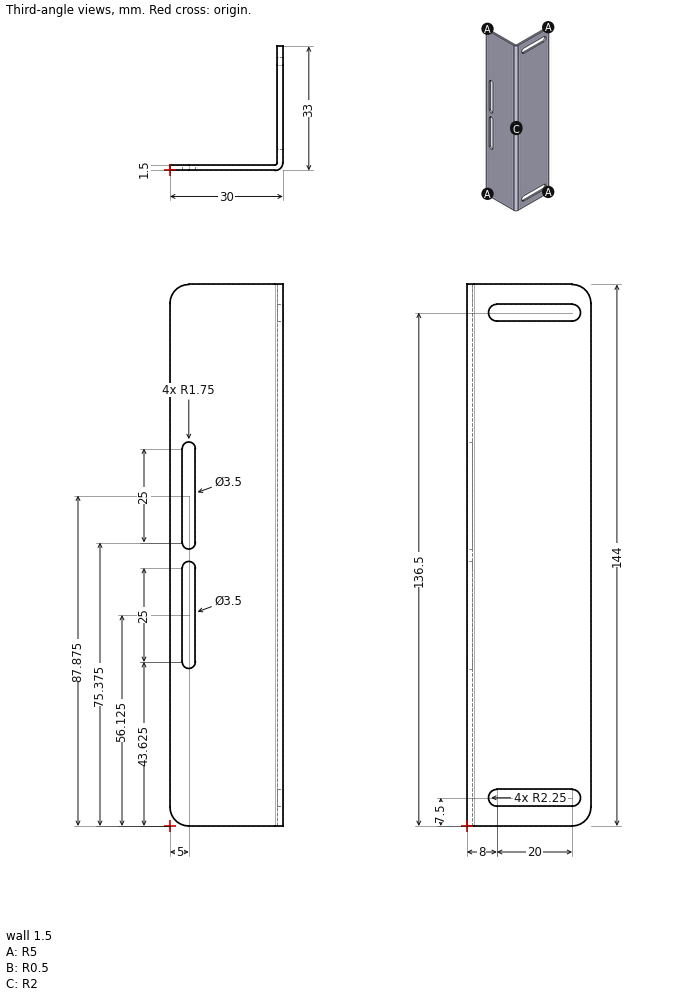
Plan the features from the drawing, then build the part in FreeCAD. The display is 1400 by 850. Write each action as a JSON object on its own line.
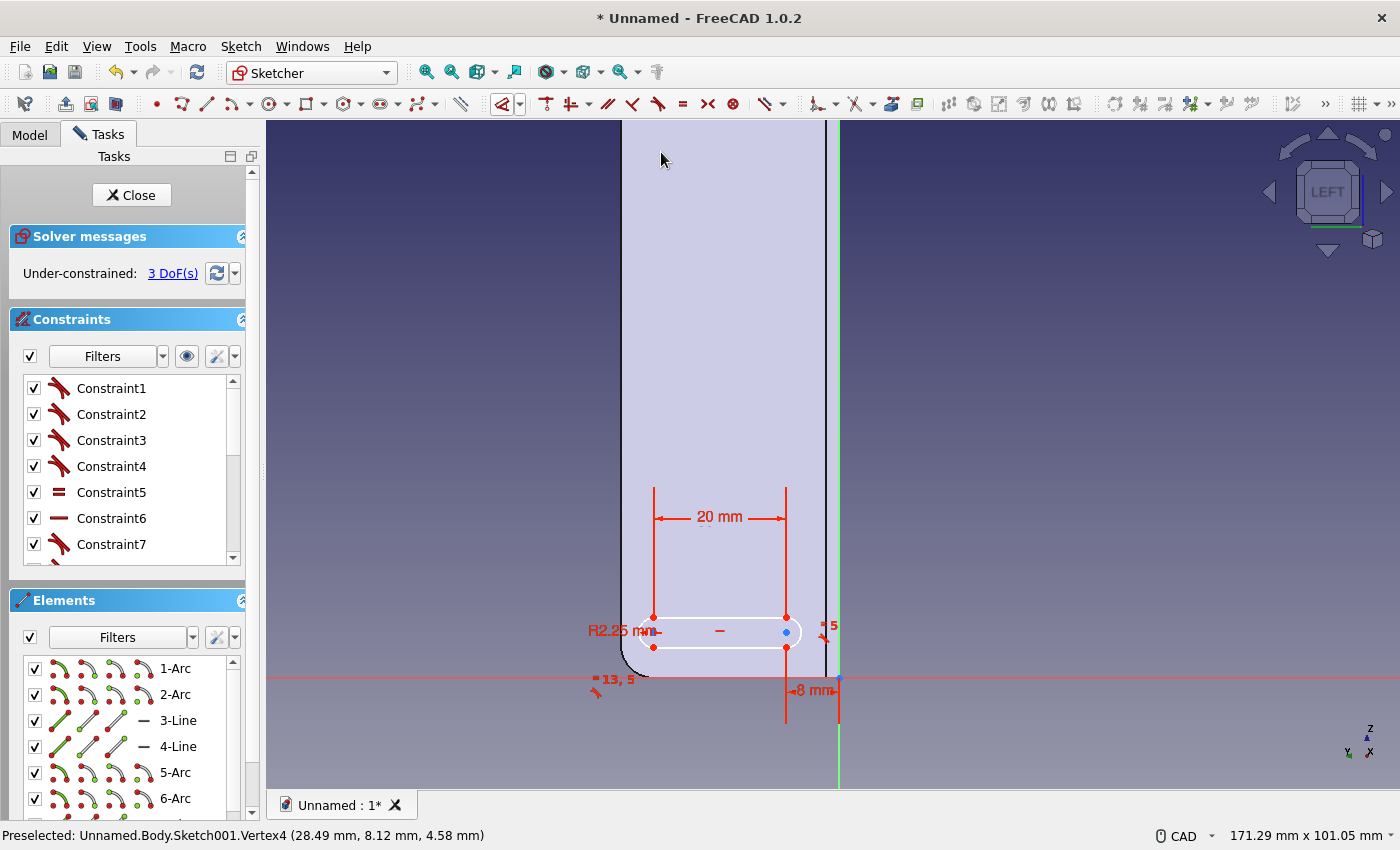
{"action": "scroll", "coordinate": [785, 647], "scroll_direction": "down", "scroll_amount": 4}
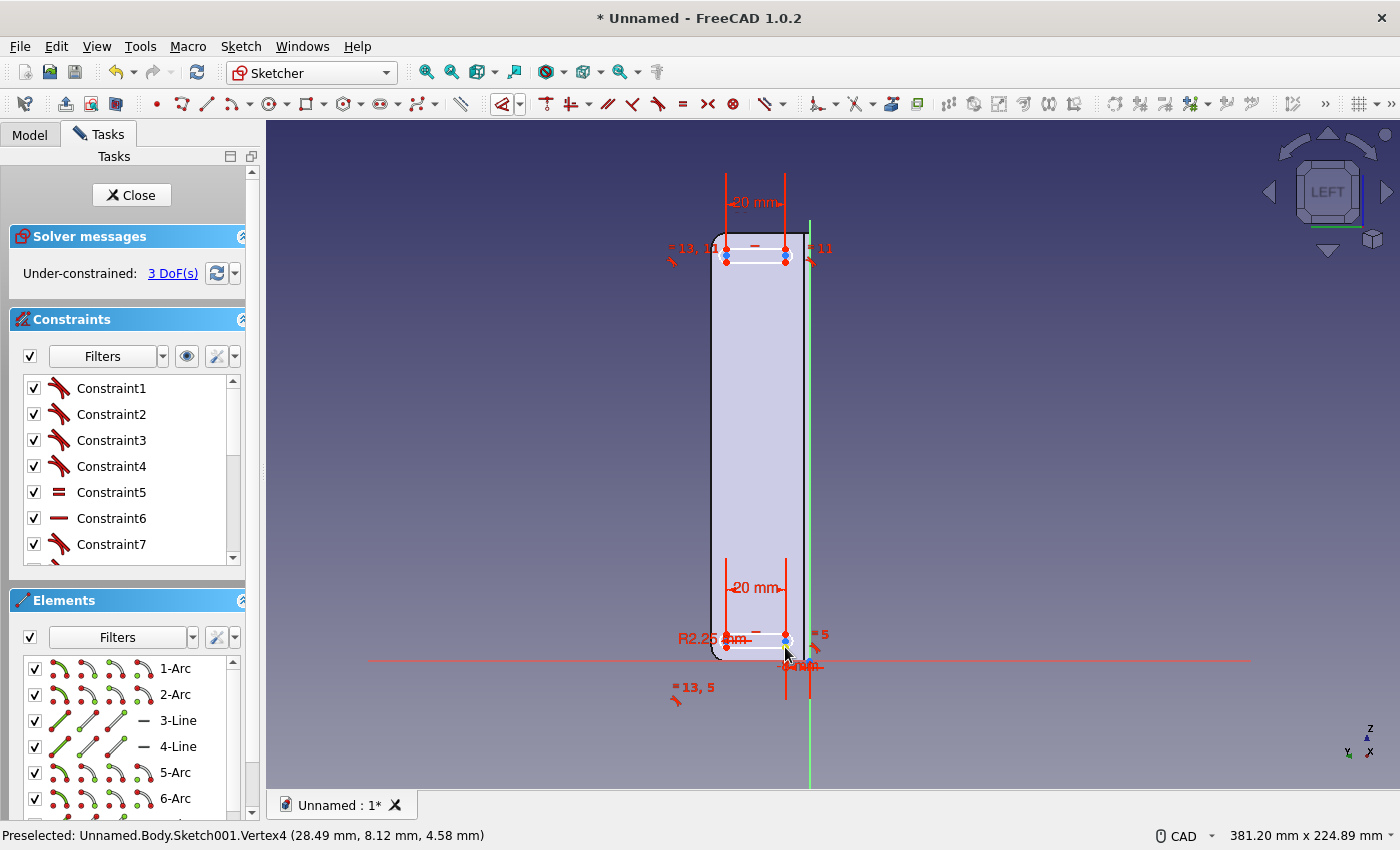
{"action": "scroll", "coordinate": [785, 263], "scroll_direction": "up", "scroll_amount": 4}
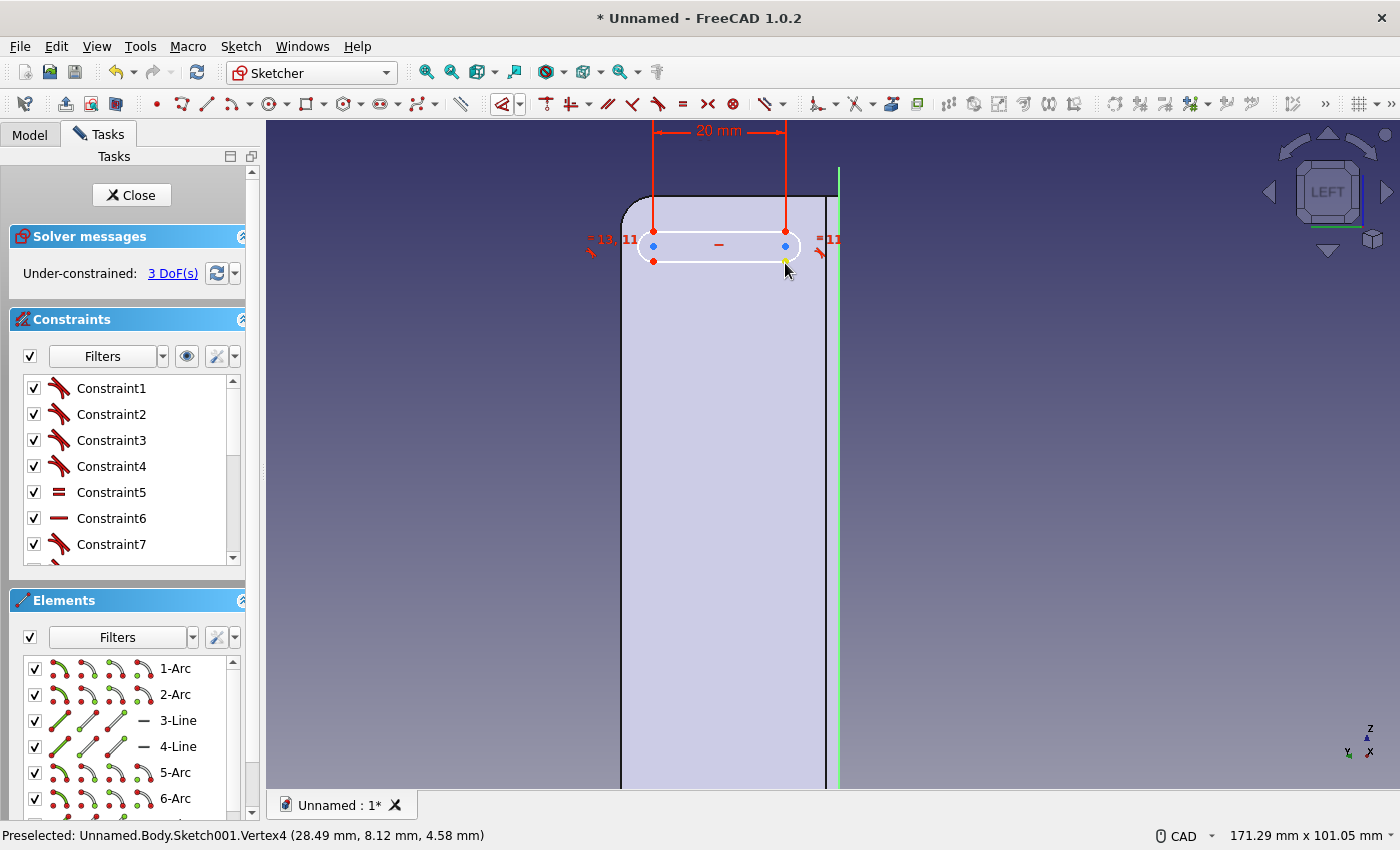
{"action": "left_click", "coordinate": [786, 262]}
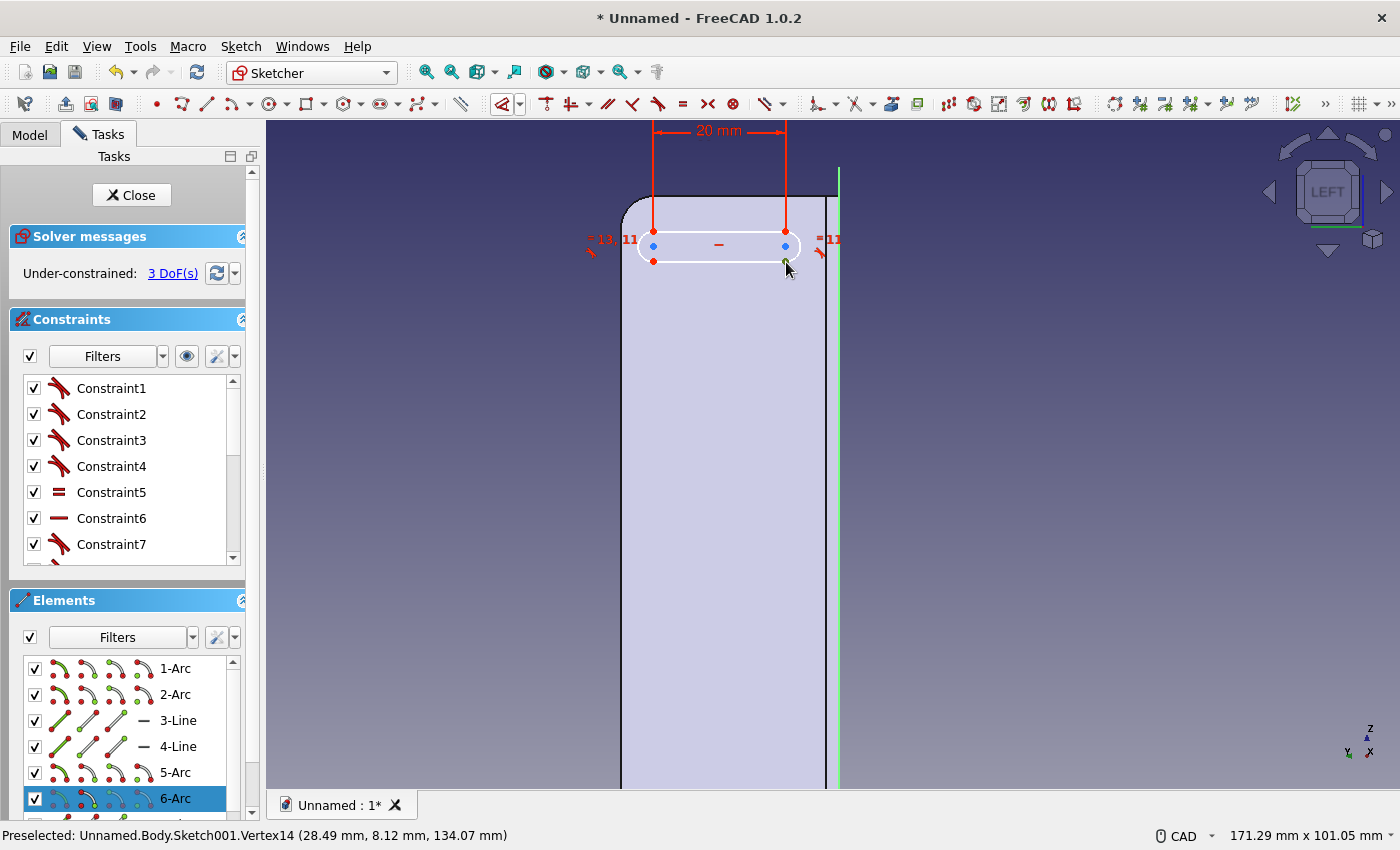
{"action": "key", "text": "l"}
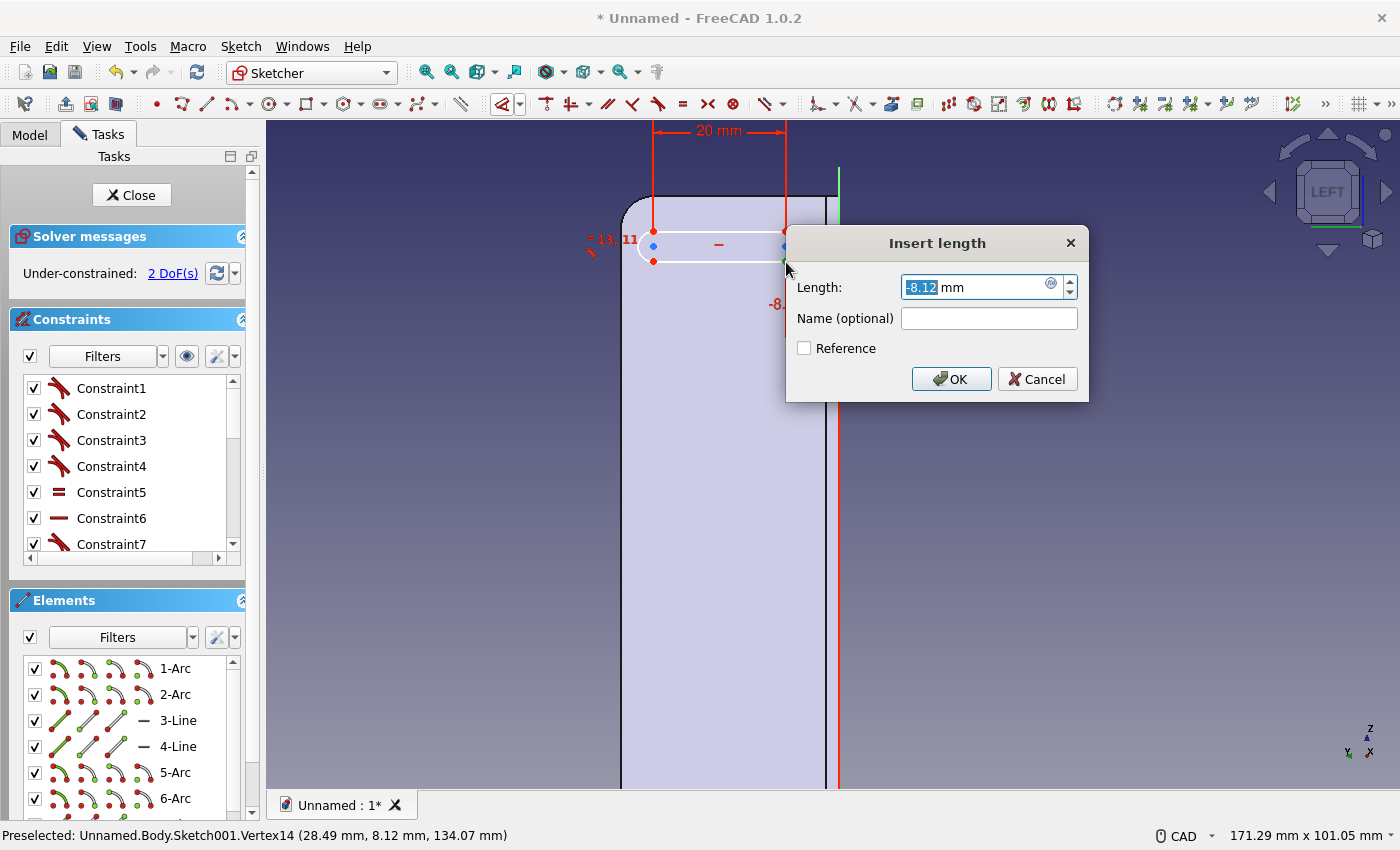
{"action": "type", "text": "-8"}
{"action": "key", "text": "Return"}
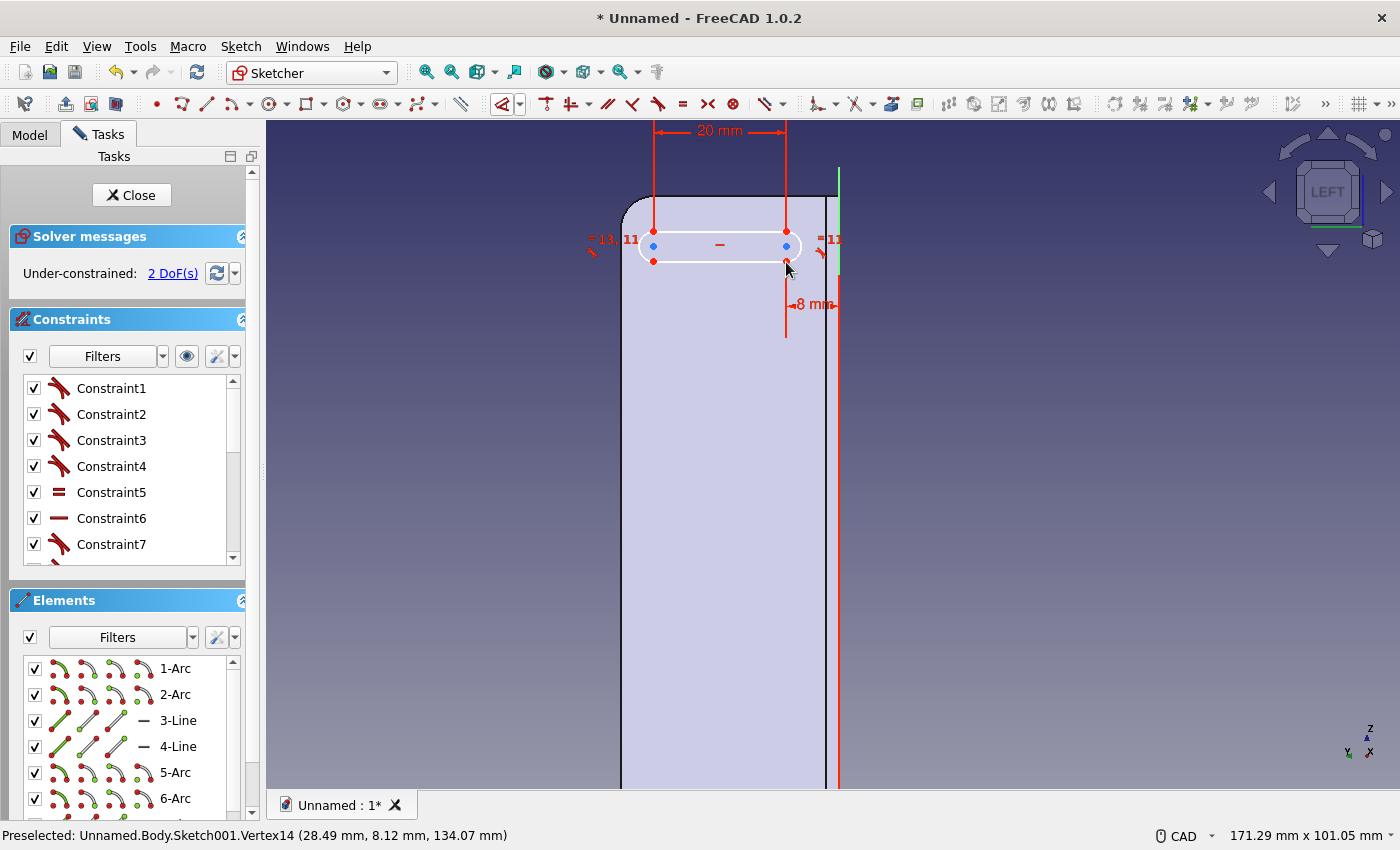
{"action": "scroll", "coordinate": [785, 262], "scroll_direction": "down", "scroll_amount": 4}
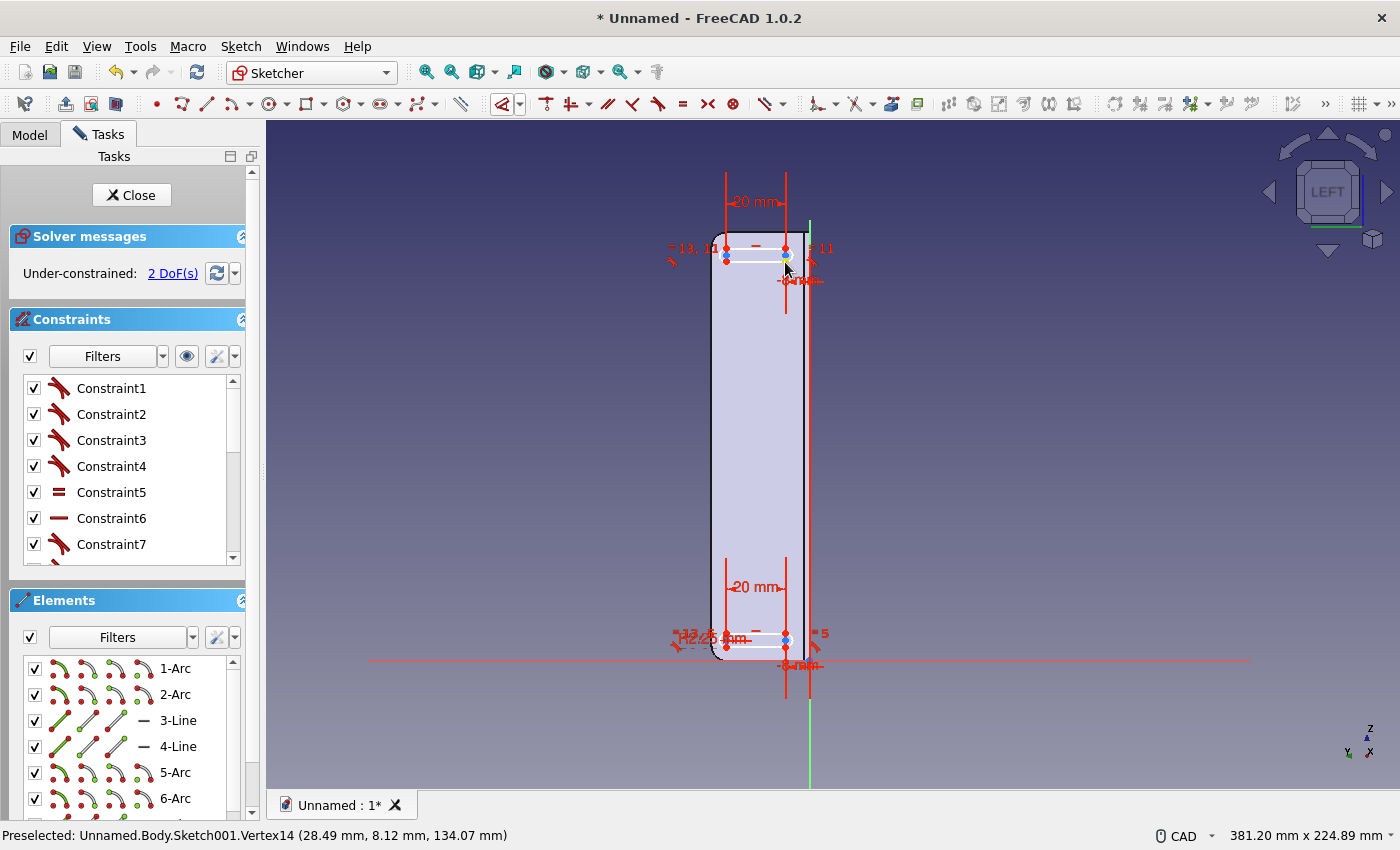
{"action": "scroll", "coordinate": [726, 641], "scroll_direction": "up", "scroll_amount": 4}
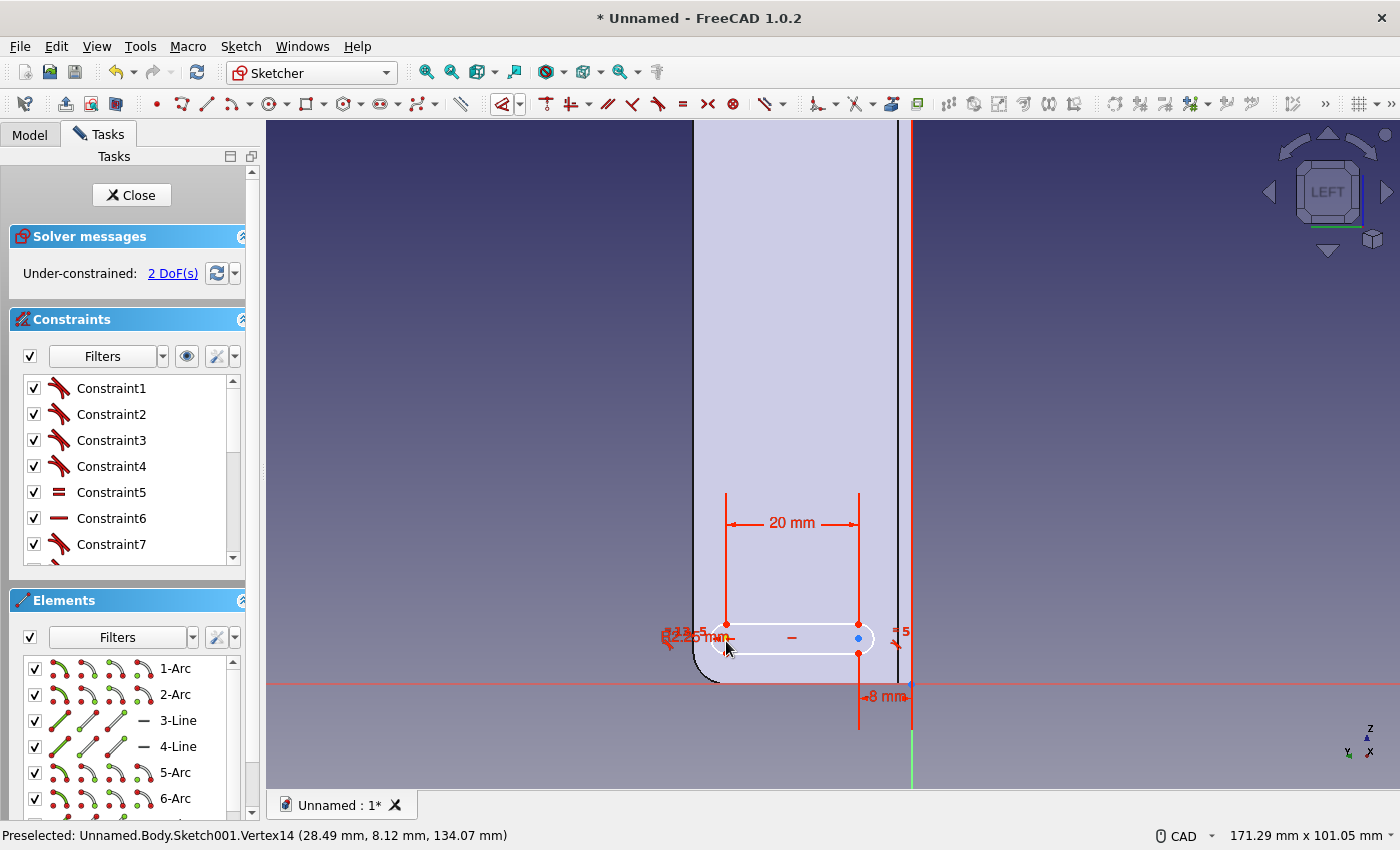
{"action": "left_click", "coordinate": [726, 639]}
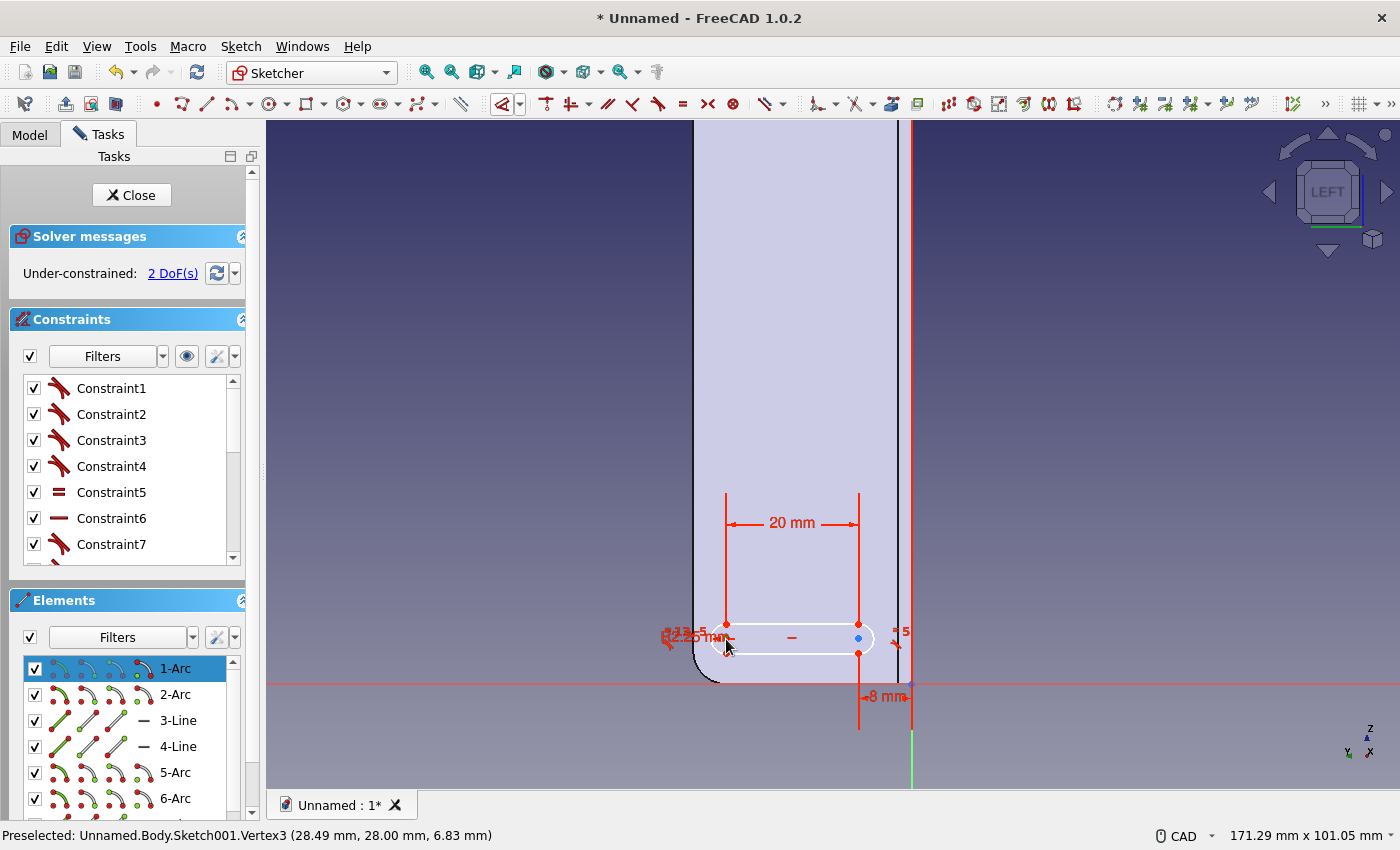
{"action": "key", "text": "i"}